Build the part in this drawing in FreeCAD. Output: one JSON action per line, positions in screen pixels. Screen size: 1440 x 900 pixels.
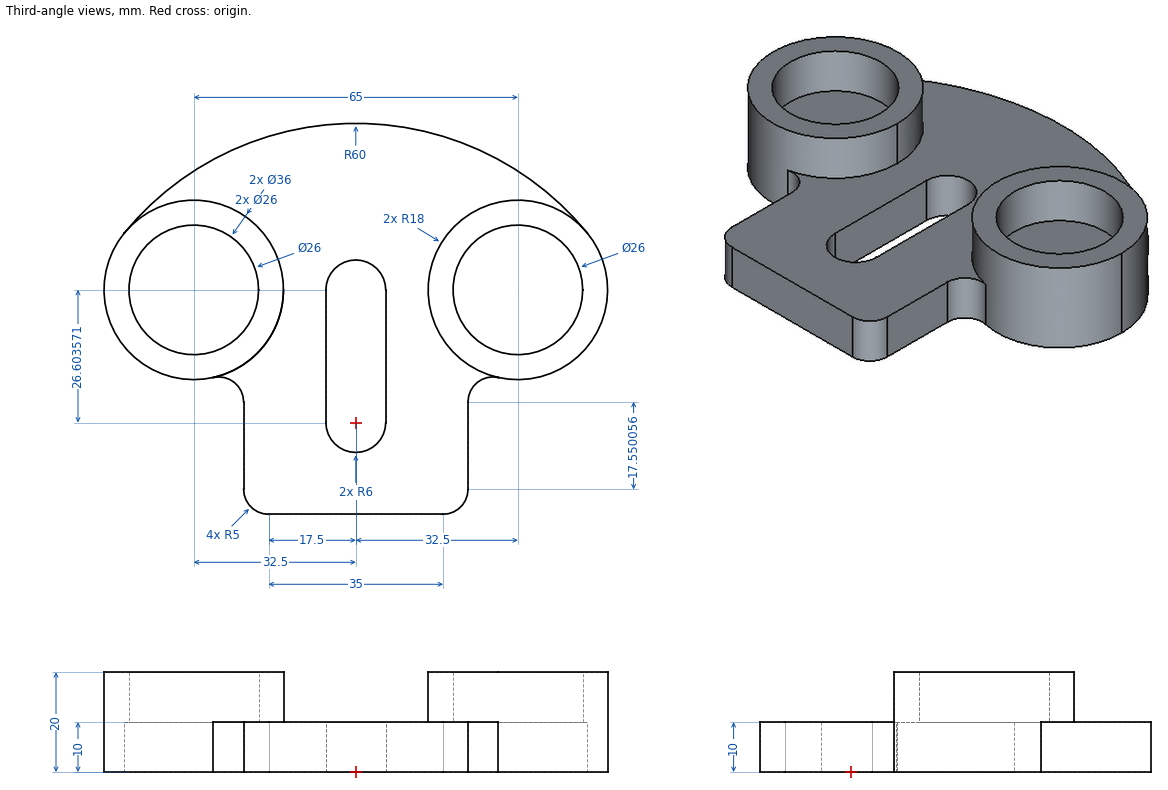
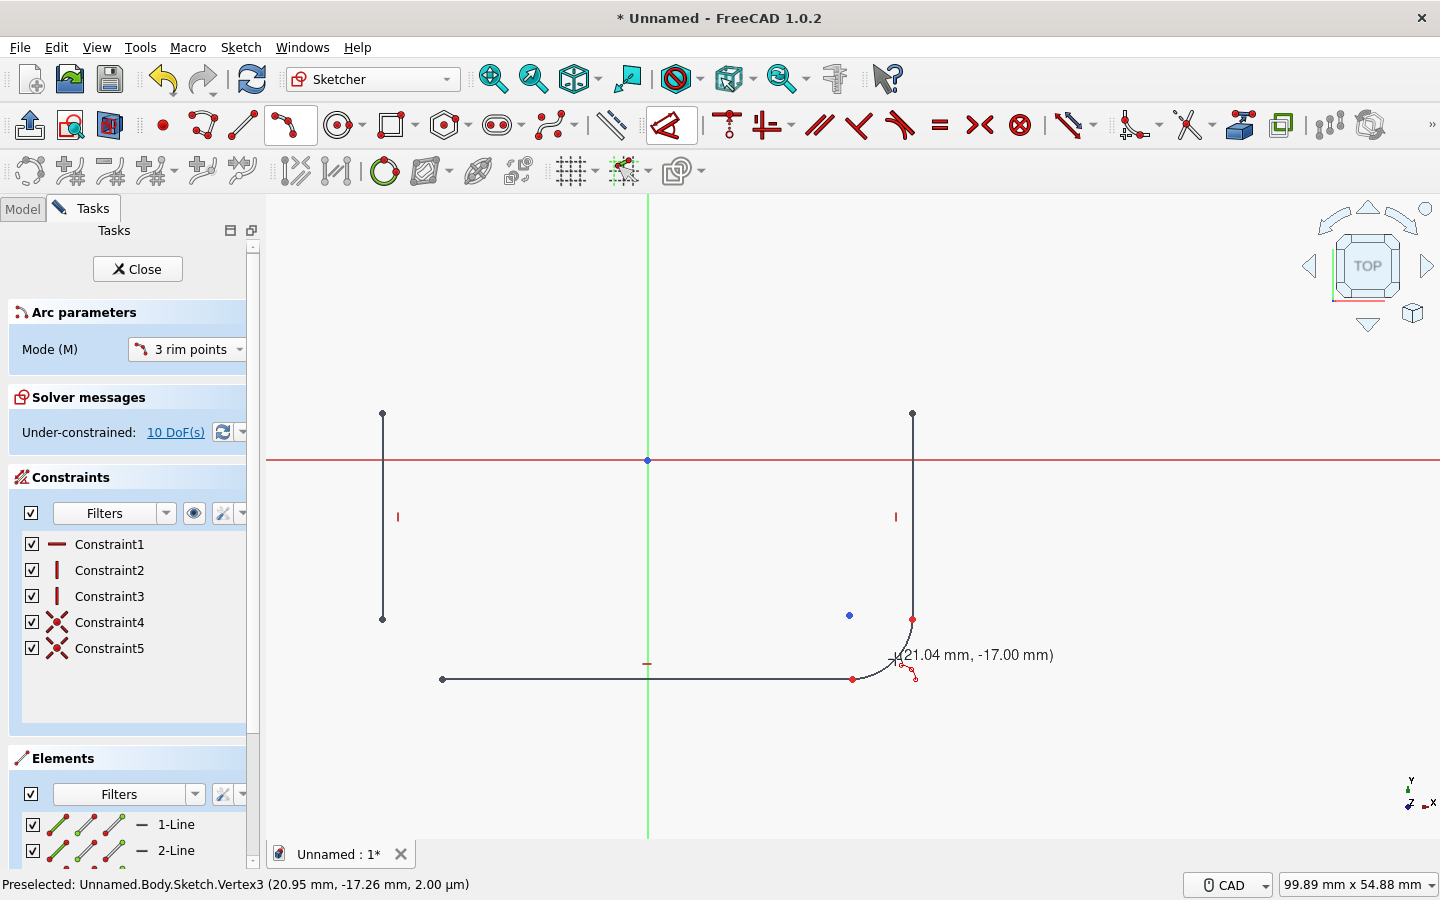
{"action": "left_click", "coordinate": [913, 413]}
{"action": "left_click", "coordinate": [984, 354]}
{"action": "left_click", "coordinate": [934, 366]}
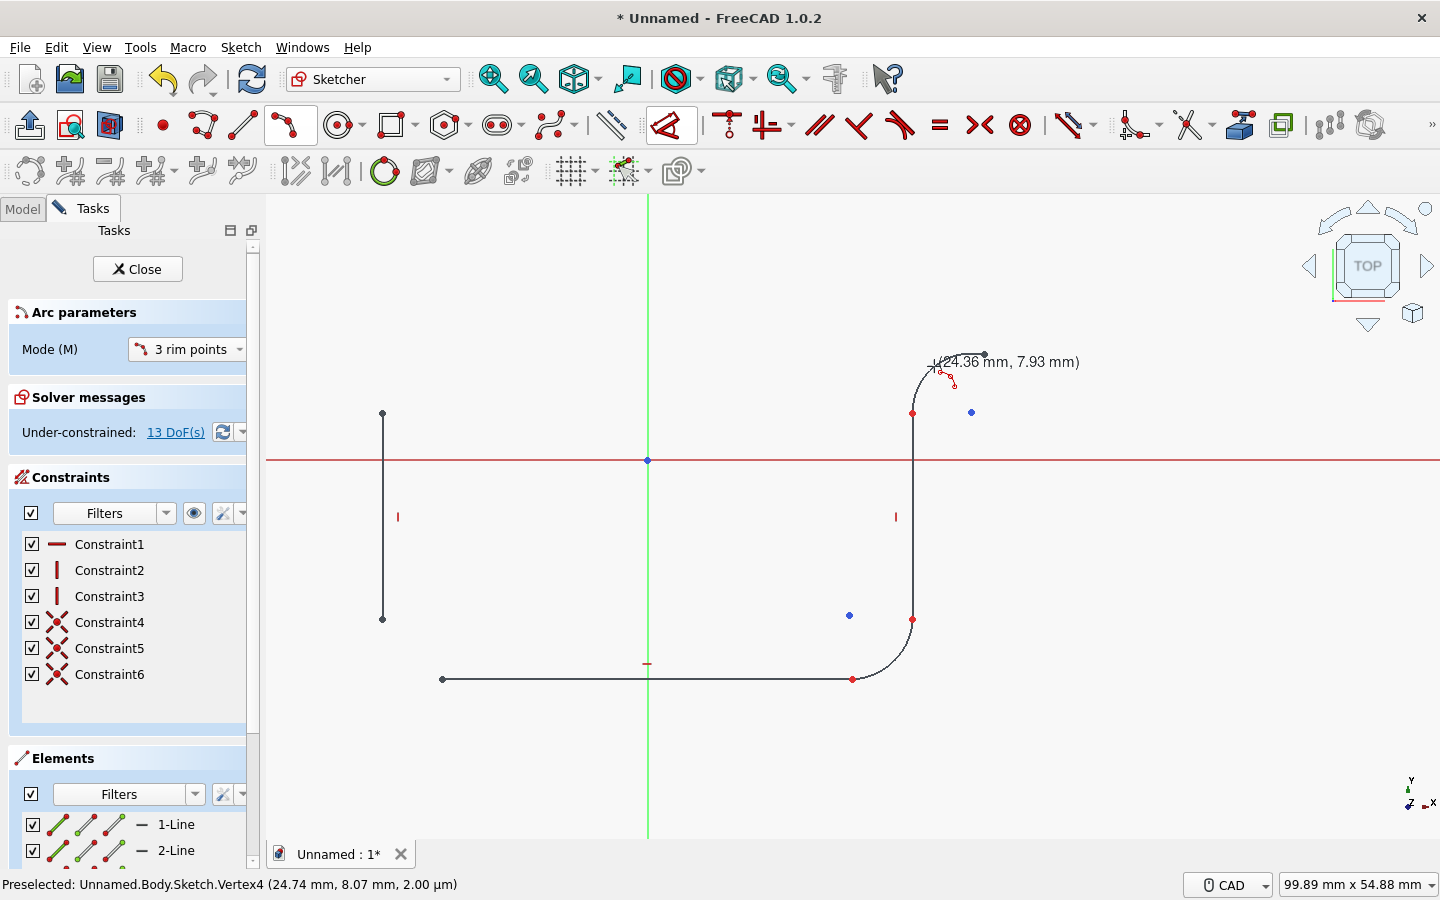
{"action": "left_click", "coordinate": [984, 355]}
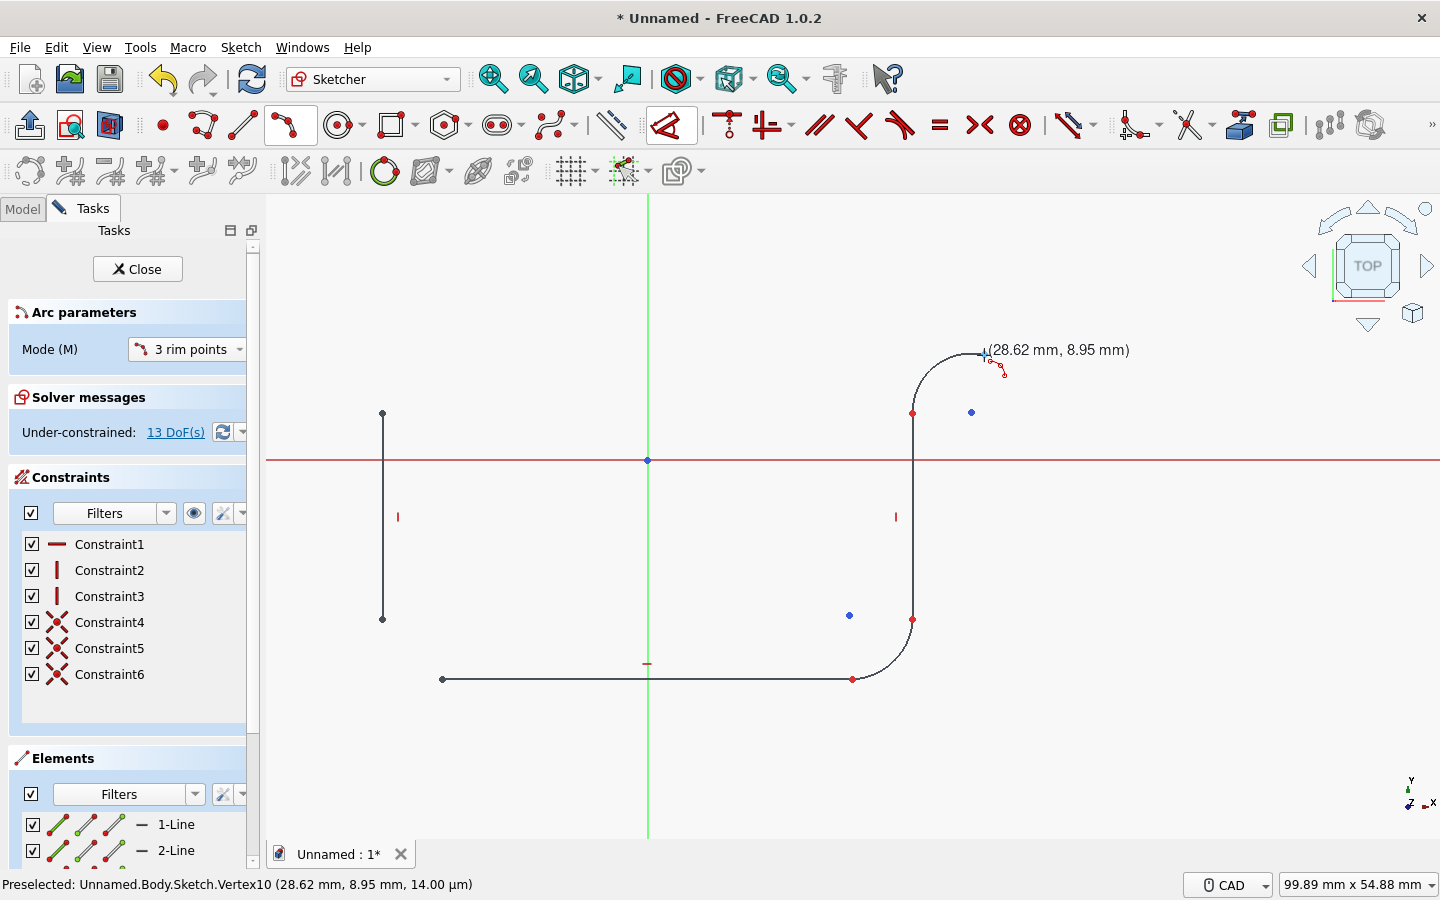
{"action": "scroll", "coordinate": [896, 762], "scroll_direction": "down", "scroll_amount": 4}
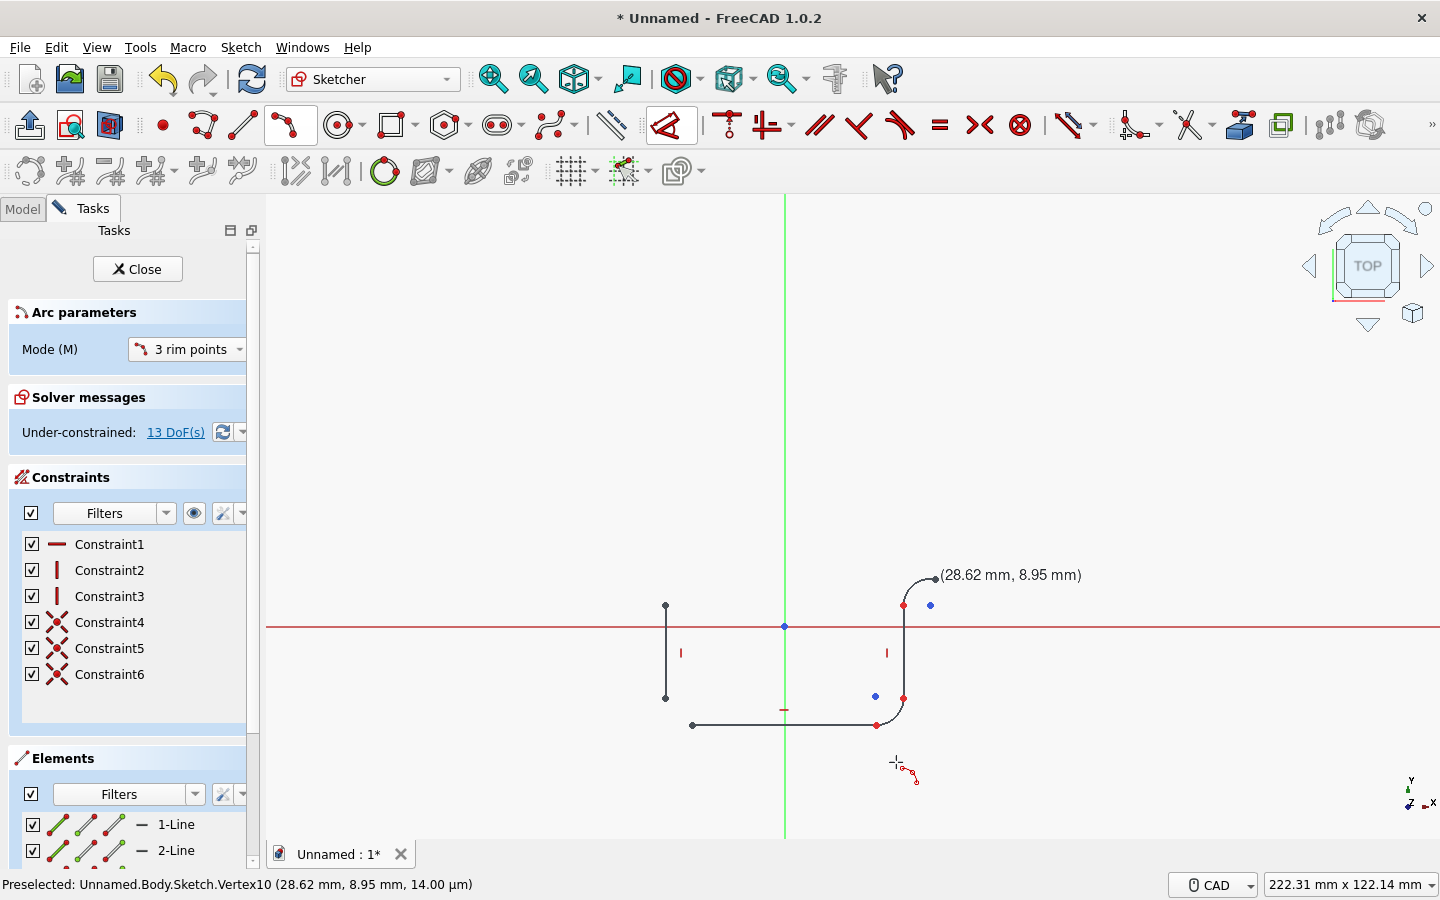
{"action": "left_click", "coordinate": [1030, 426]}
{"action": "left_click", "coordinate": [875, 437]}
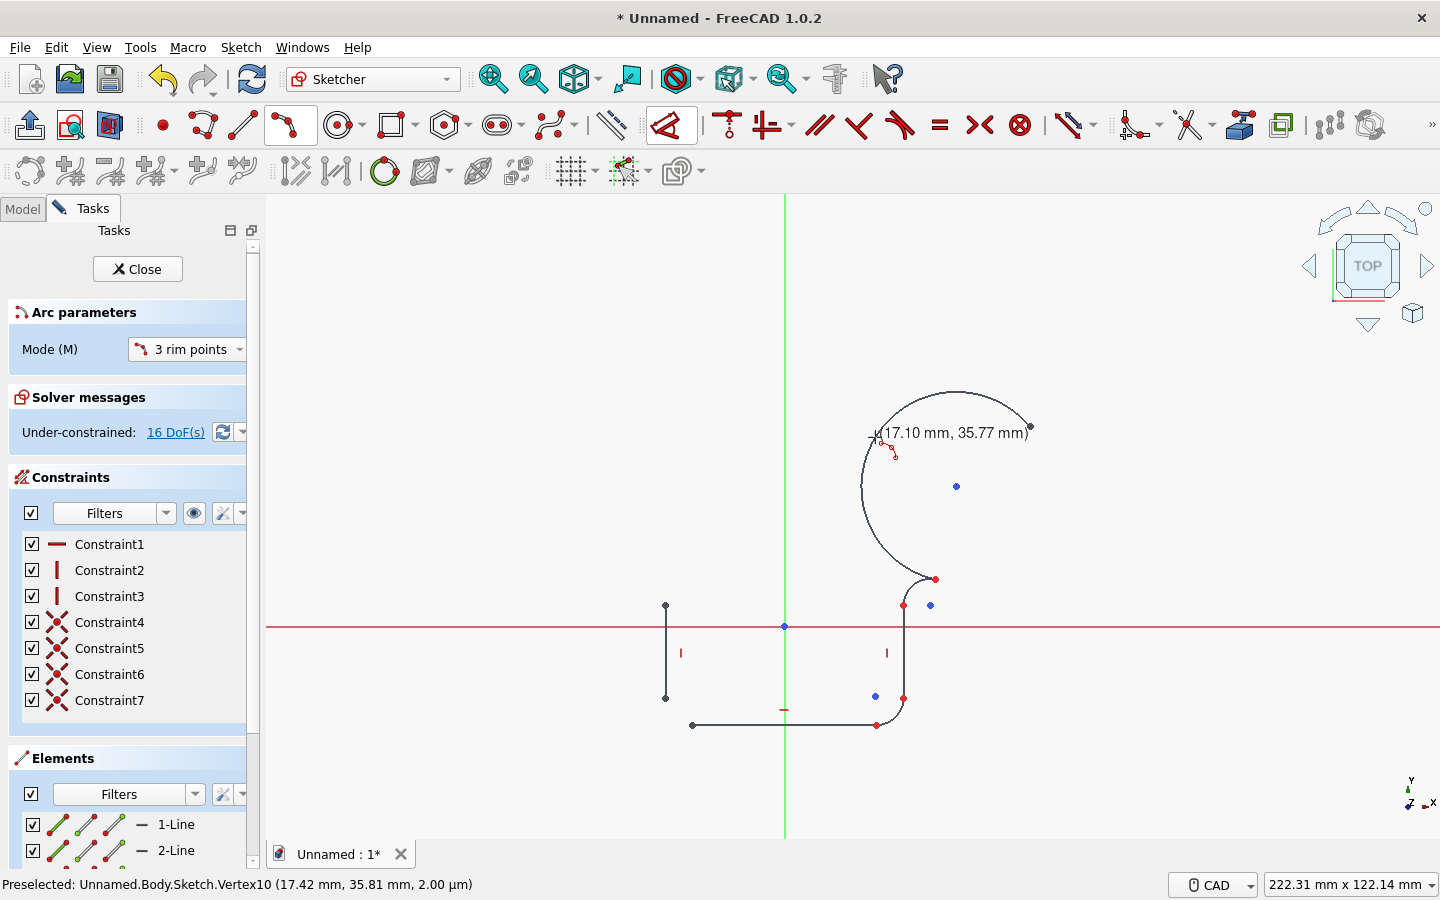
{"action": "left_click", "coordinate": [1030, 427]}
{"action": "left_click", "coordinate": [540, 426]}
{"action": "left_click", "coordinate": [841, 315]}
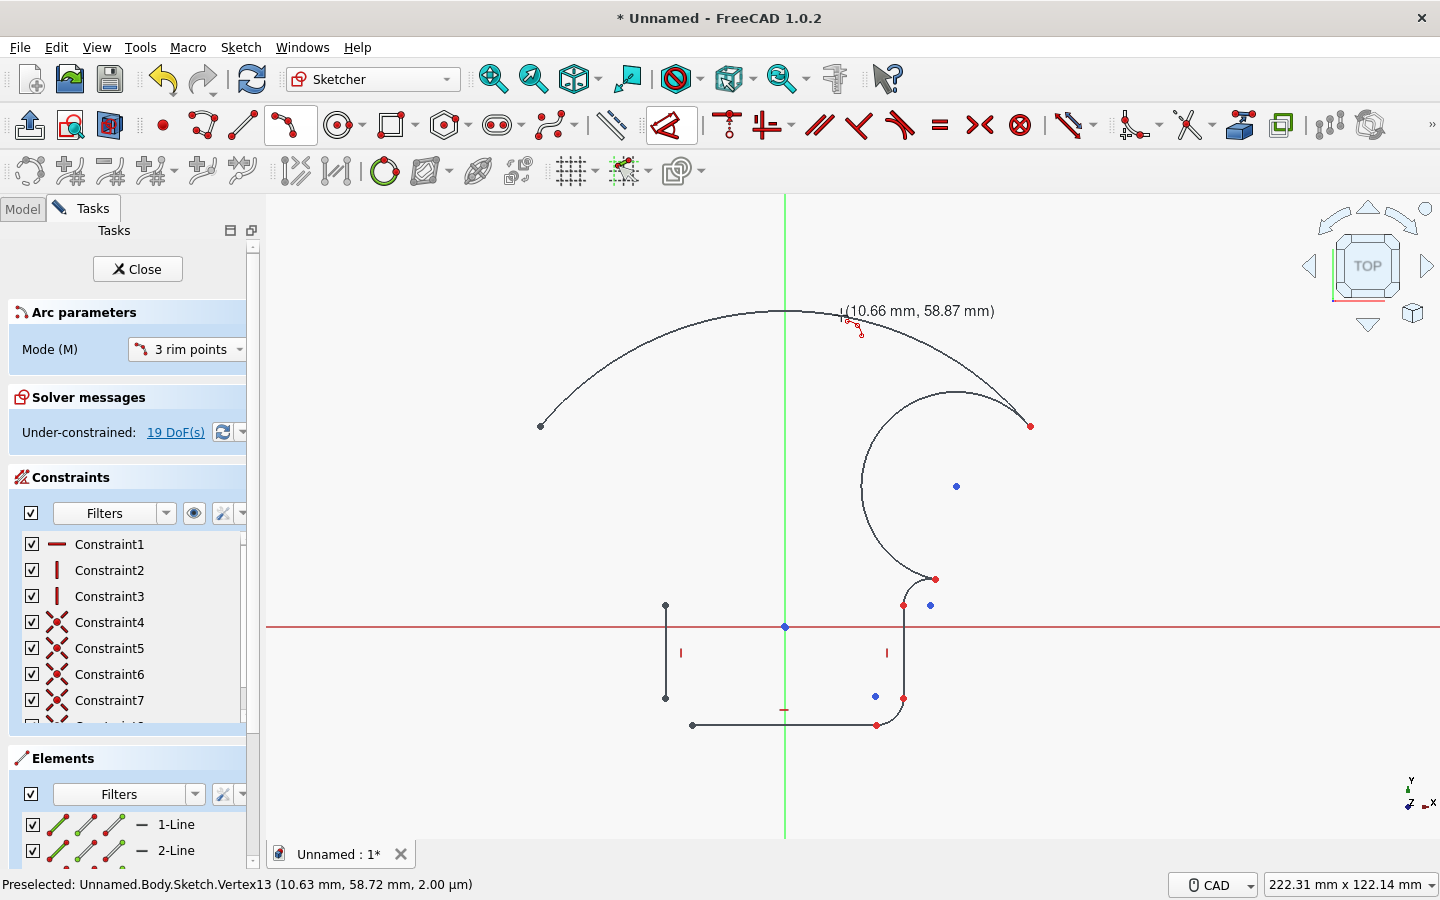
{"action": "left_click", "coordinate": [540, 427]}
{"action": "left_click", "coordinate": [634, 579]}
{"action": "left_click", "coordinate": [694, 437]}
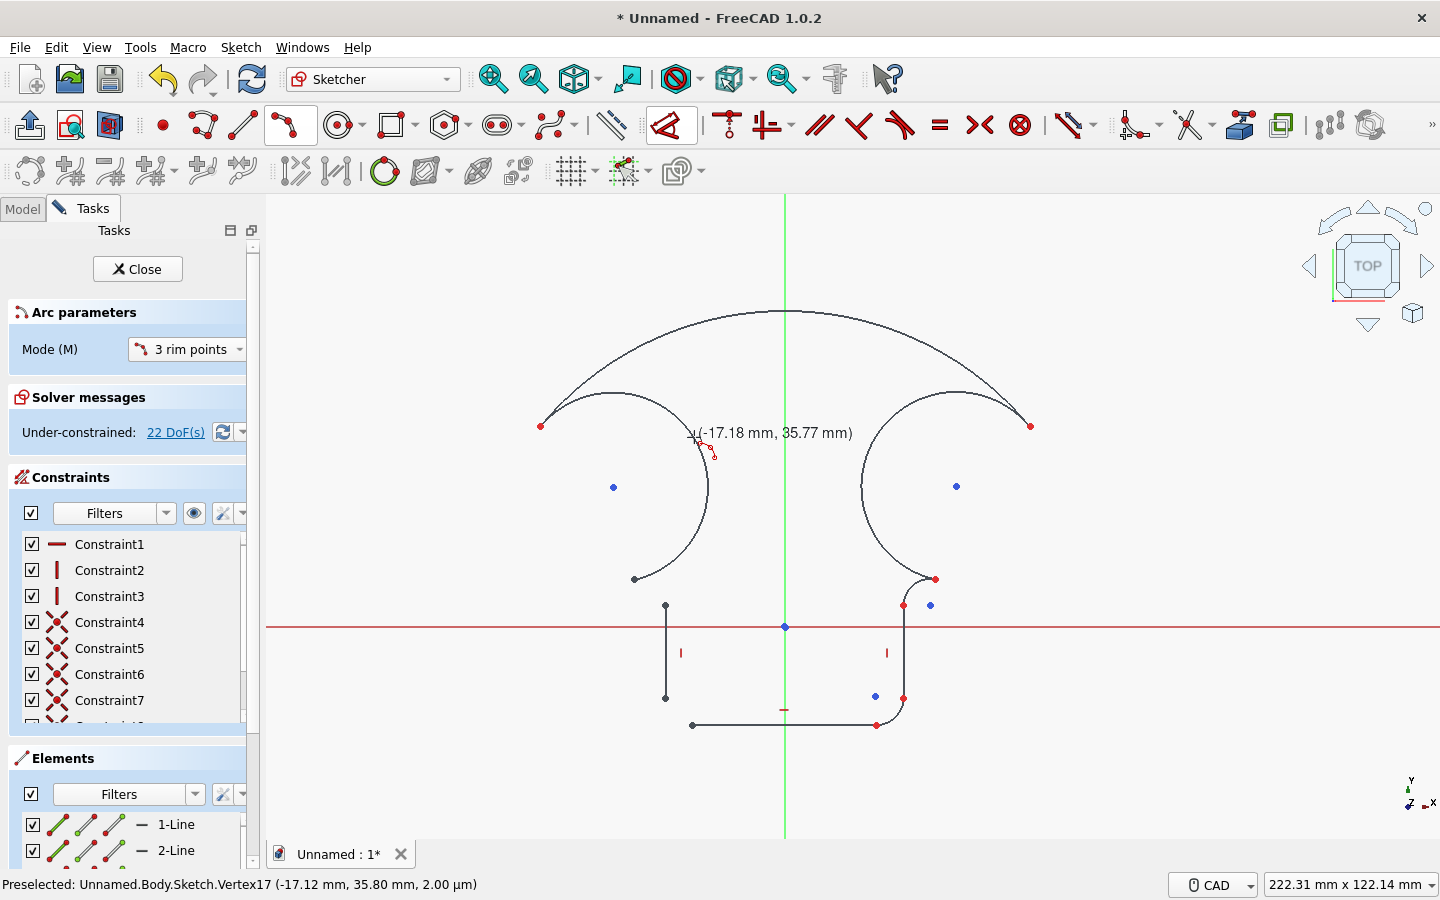
{"action": "left_click", "coordinate": [634, 580]}
{"action": "left_click", "coordinate": [666, 606]}